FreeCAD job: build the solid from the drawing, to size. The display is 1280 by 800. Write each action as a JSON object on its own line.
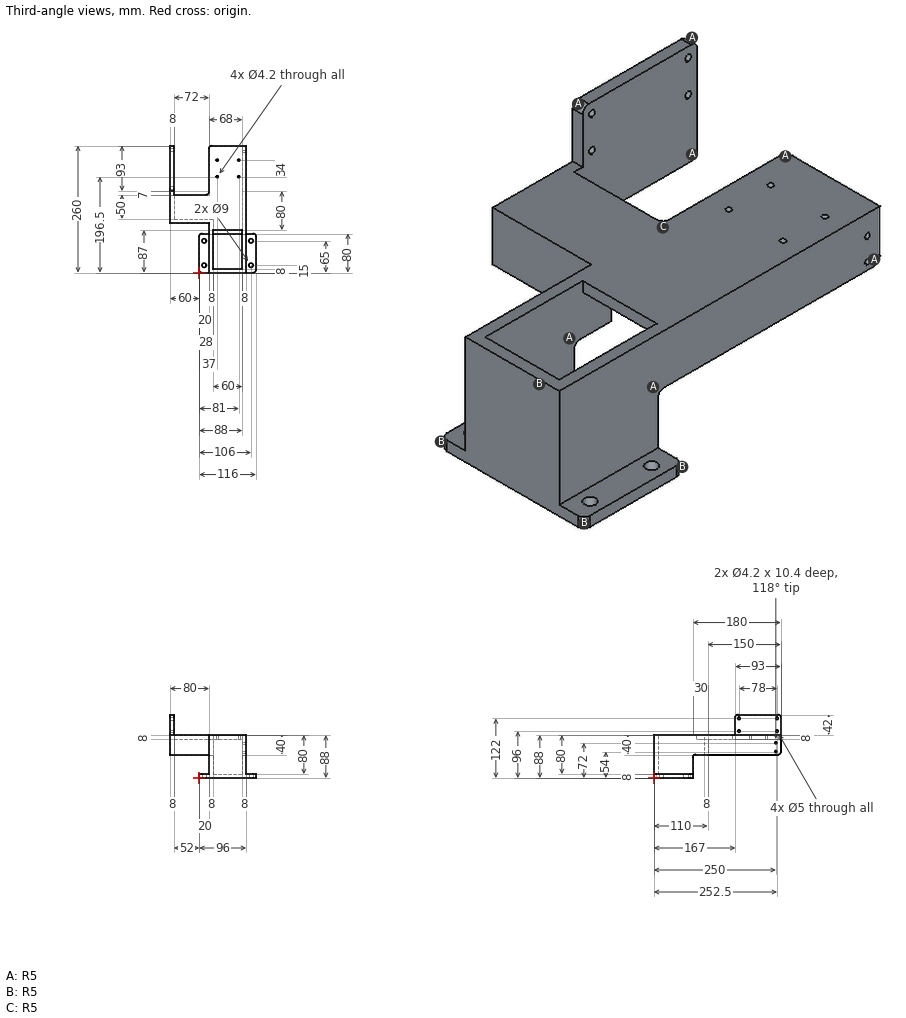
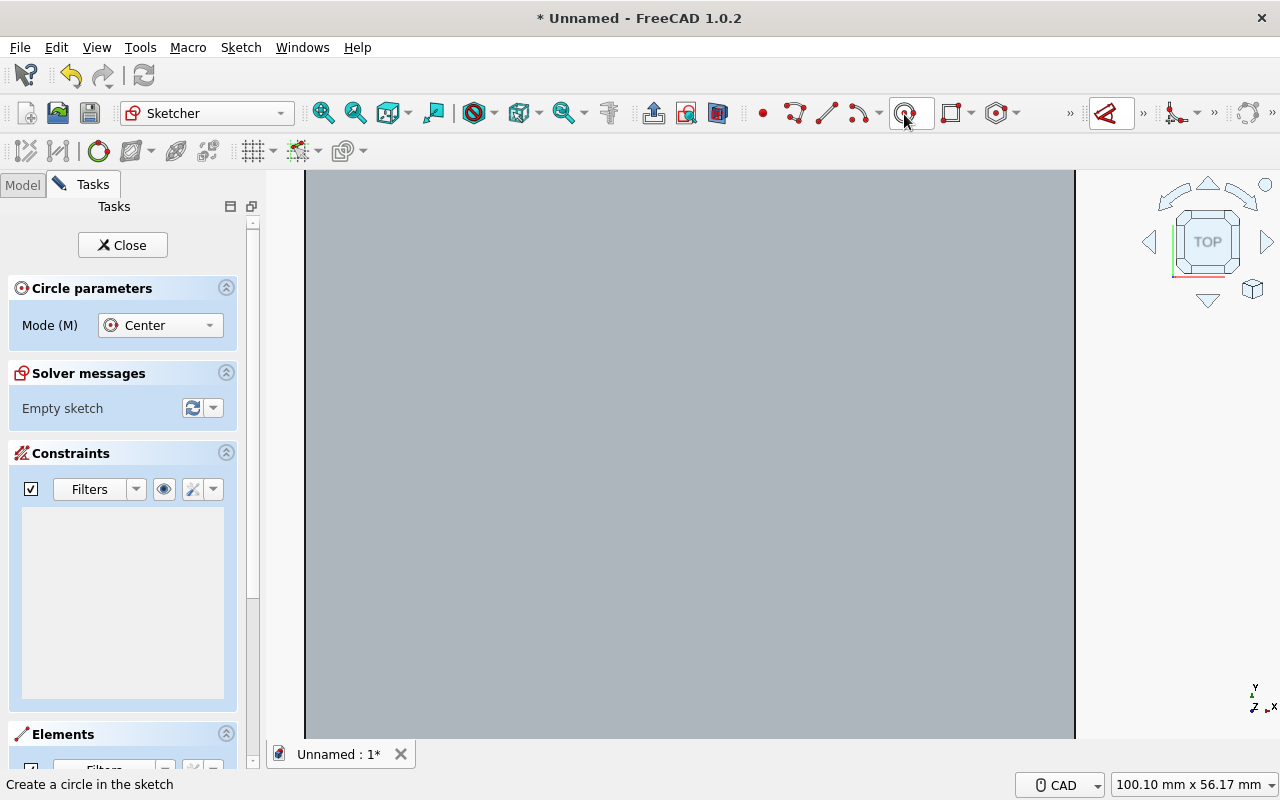
{"action": "left_click", "coordinate": [477, 626]}
{"action": "left_click", "coordinate": [493, 611]}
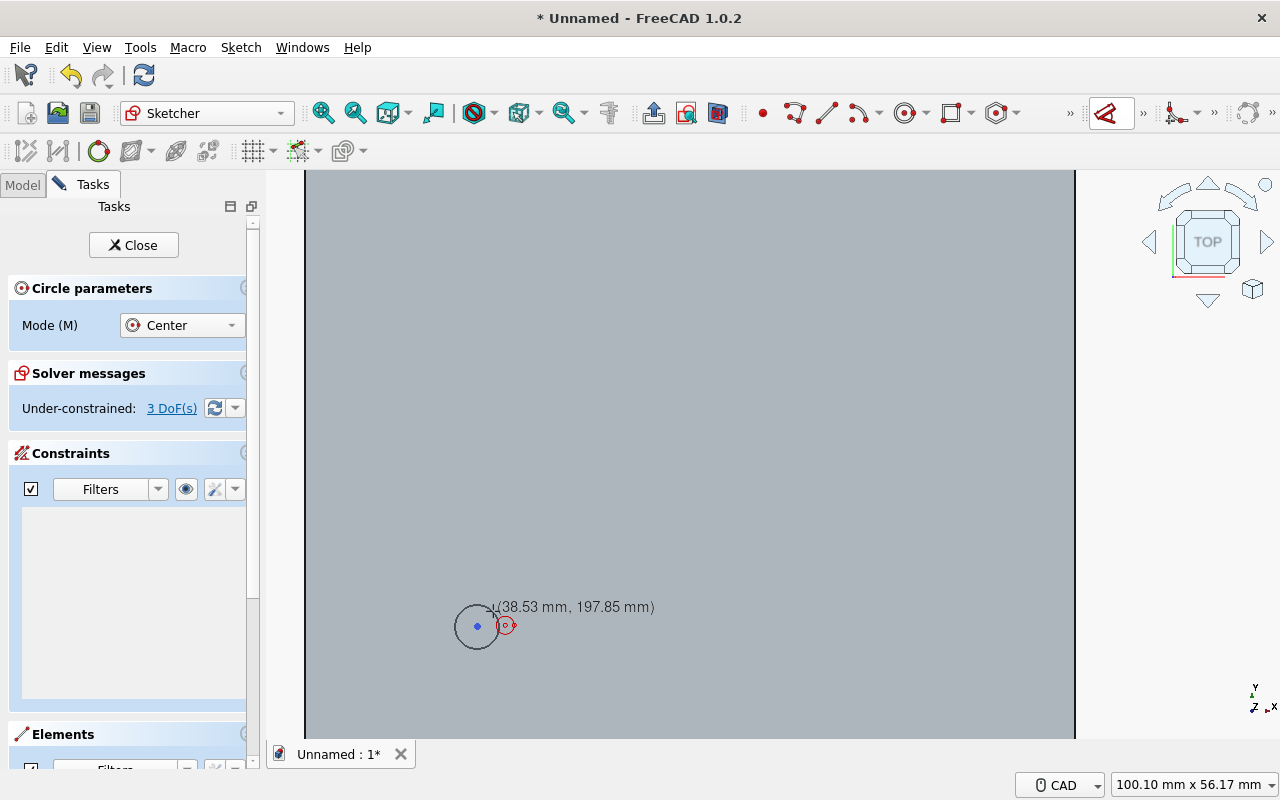
{"action": "left_click", "coordinate": [923, 626]}
{"action": "left_click", "coordinate": [938, 611]}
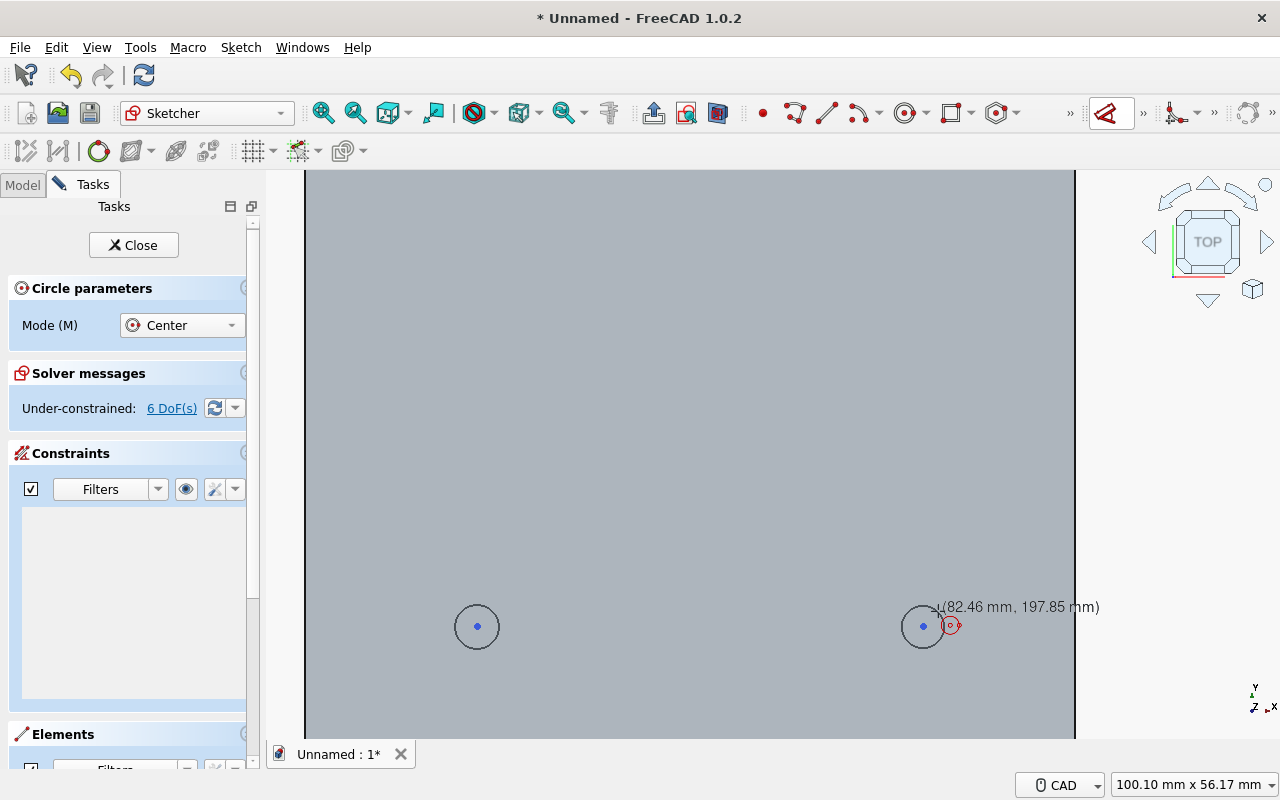
{"action": "left_click", "coordinate": [923, 281]}
{"action": "left_click", "coordinate": [938, 266]}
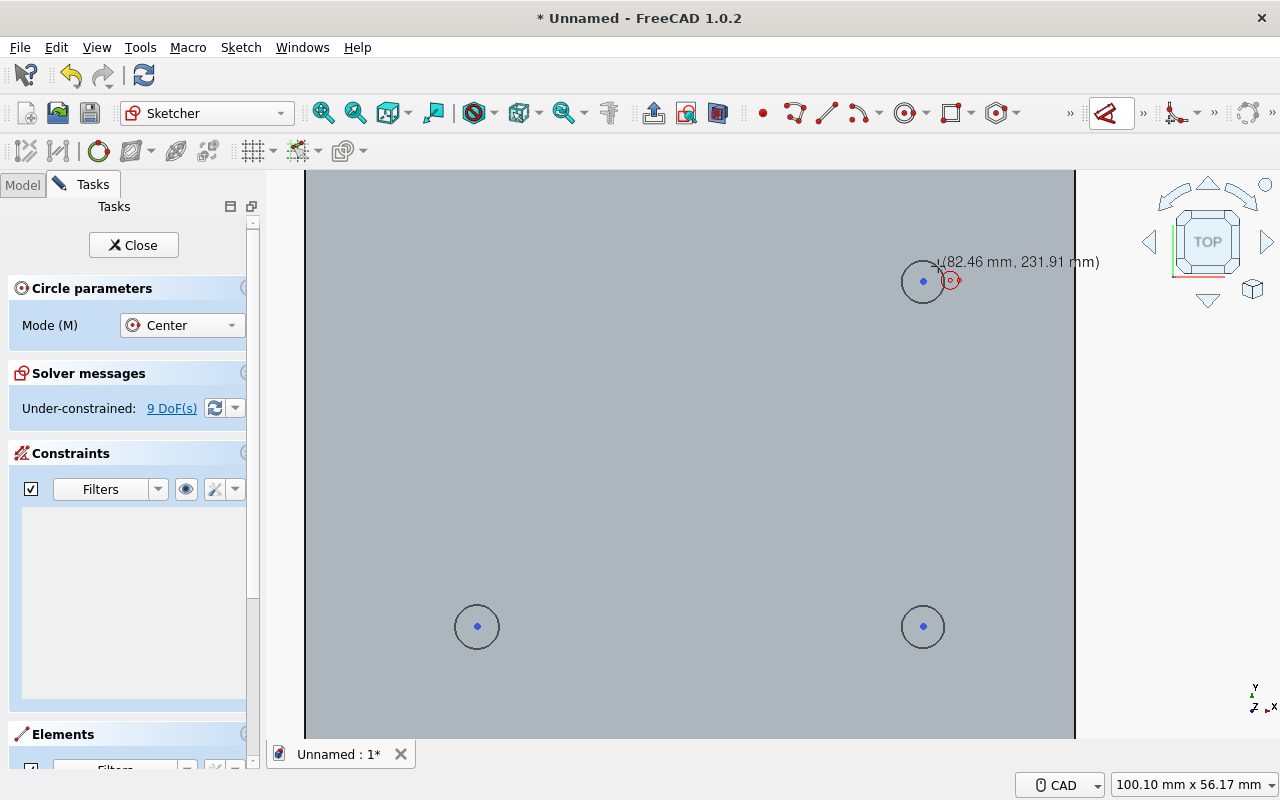
{"action": "left_click", "coordinate": [477, 281]}
{"action": "left_click", "coordinate": [493, 266]}
{"action": "key", "text": "Escape"}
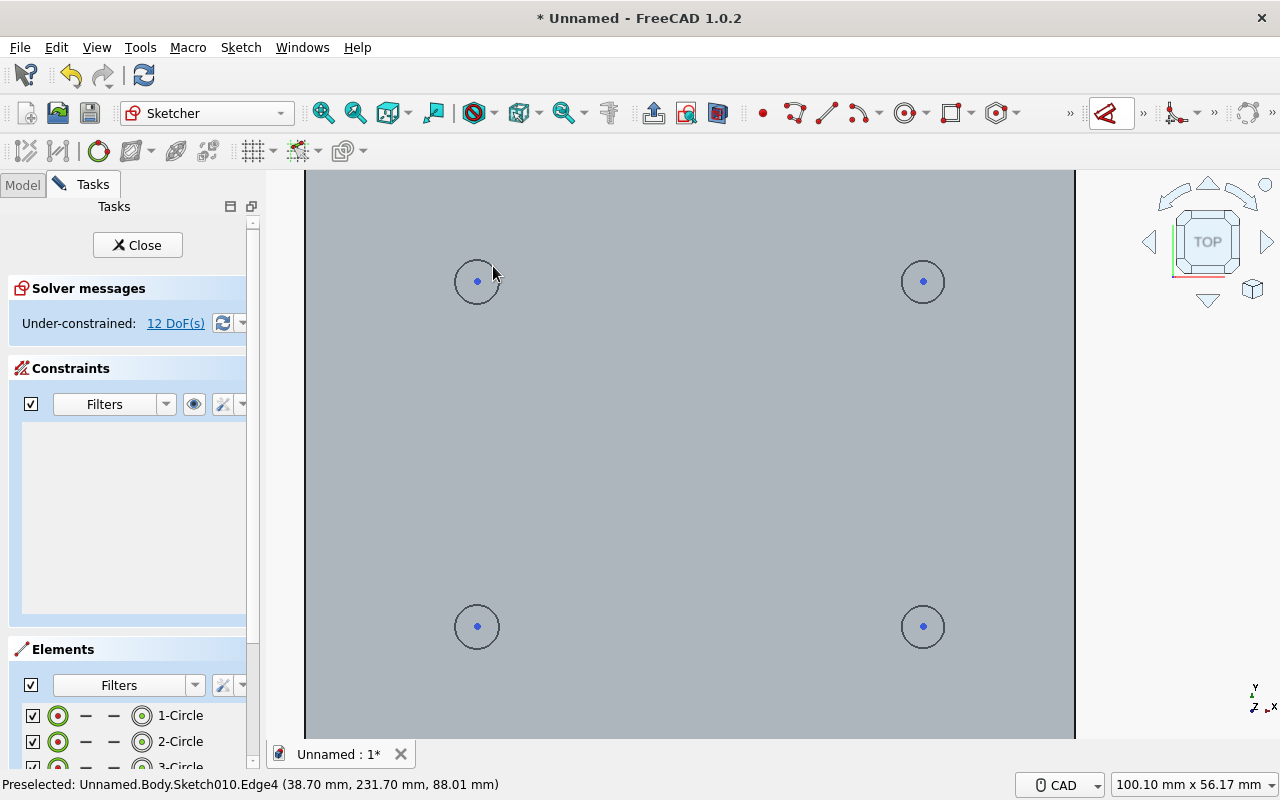
{"action": "left_click", "coordinate": [492, 611]}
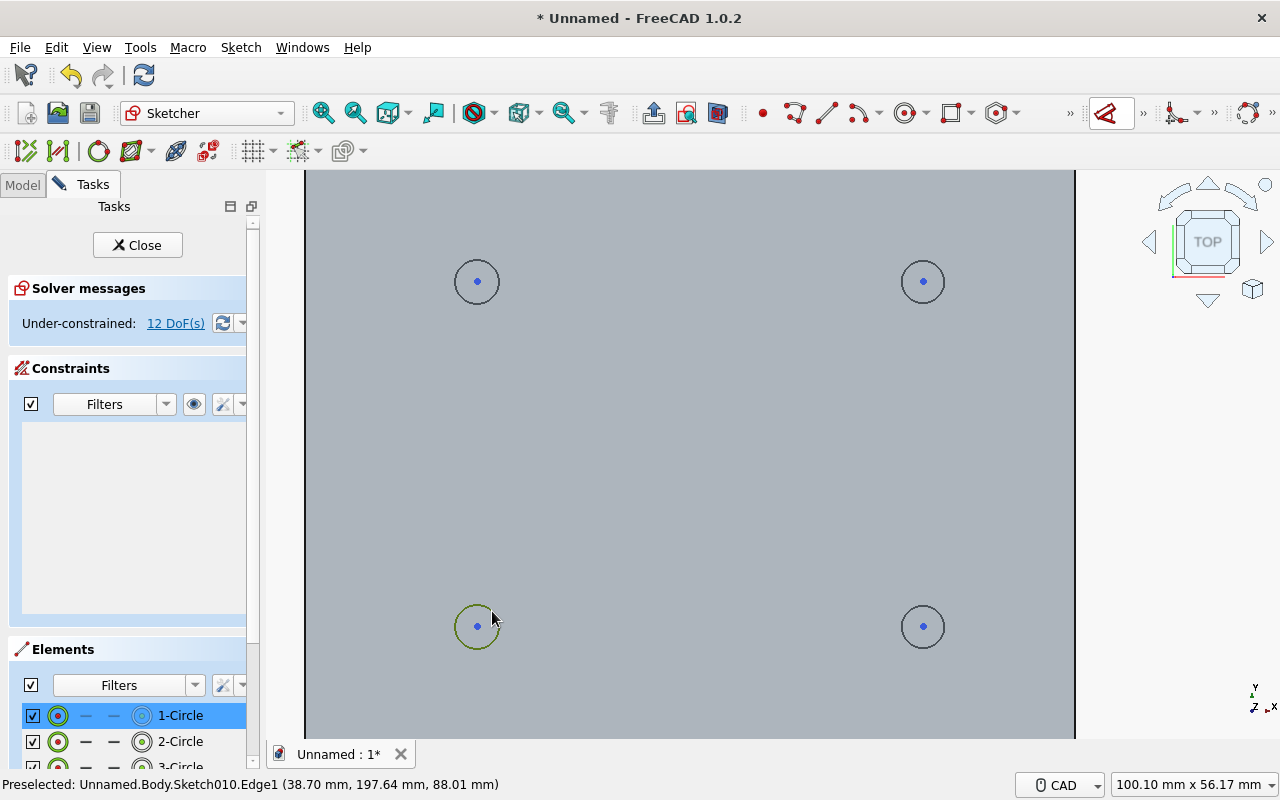
{"action": "left_click", "coordinate": [938, 612]}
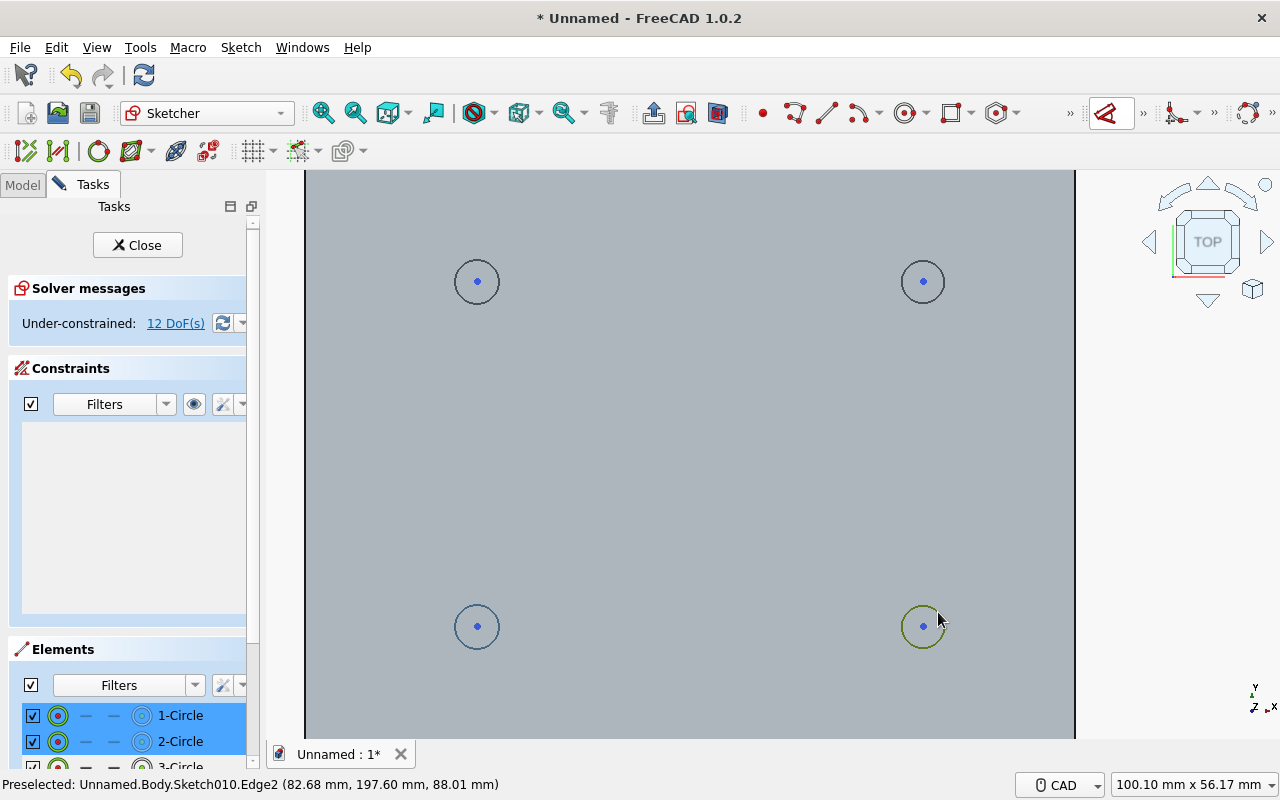
{"action": "left_click", "coordinate": [938, 267]}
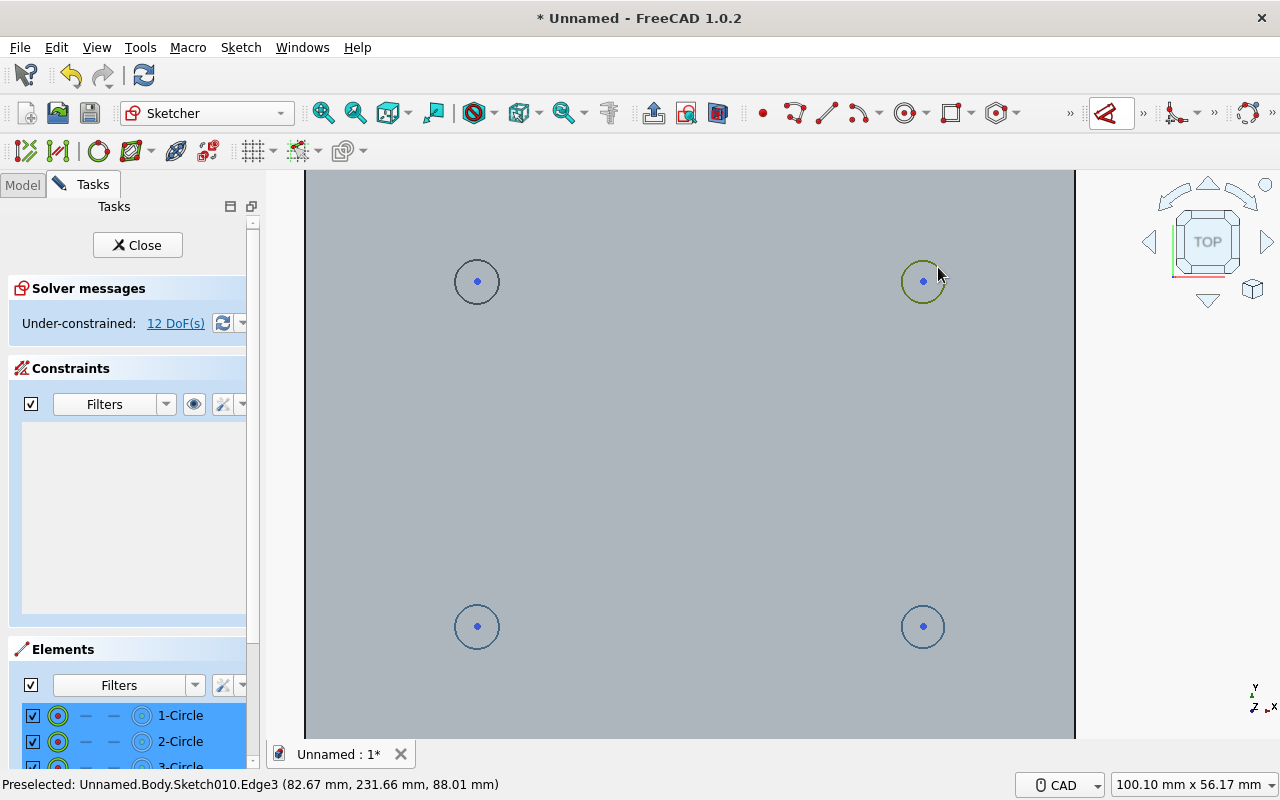
{"action": "left_click", "coordinate": [492, 266]}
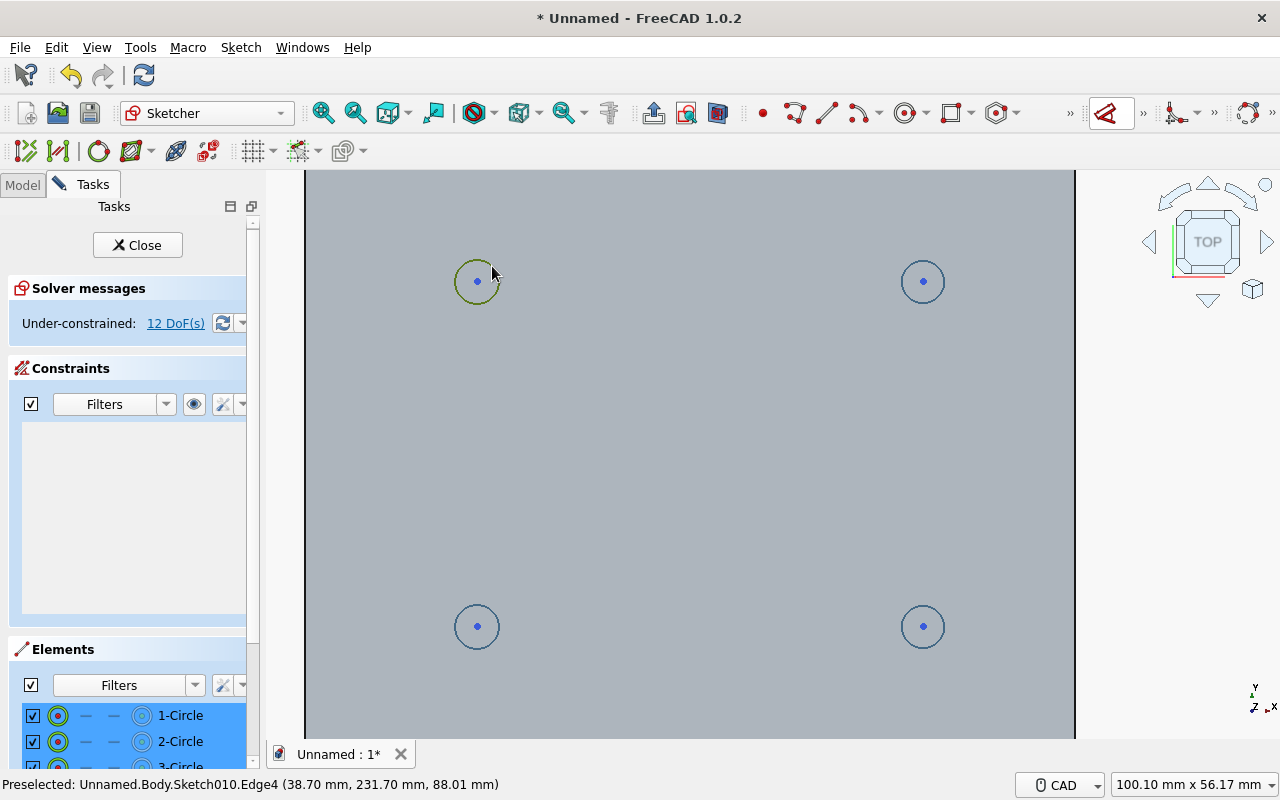
{"action": "key", "text": "e"}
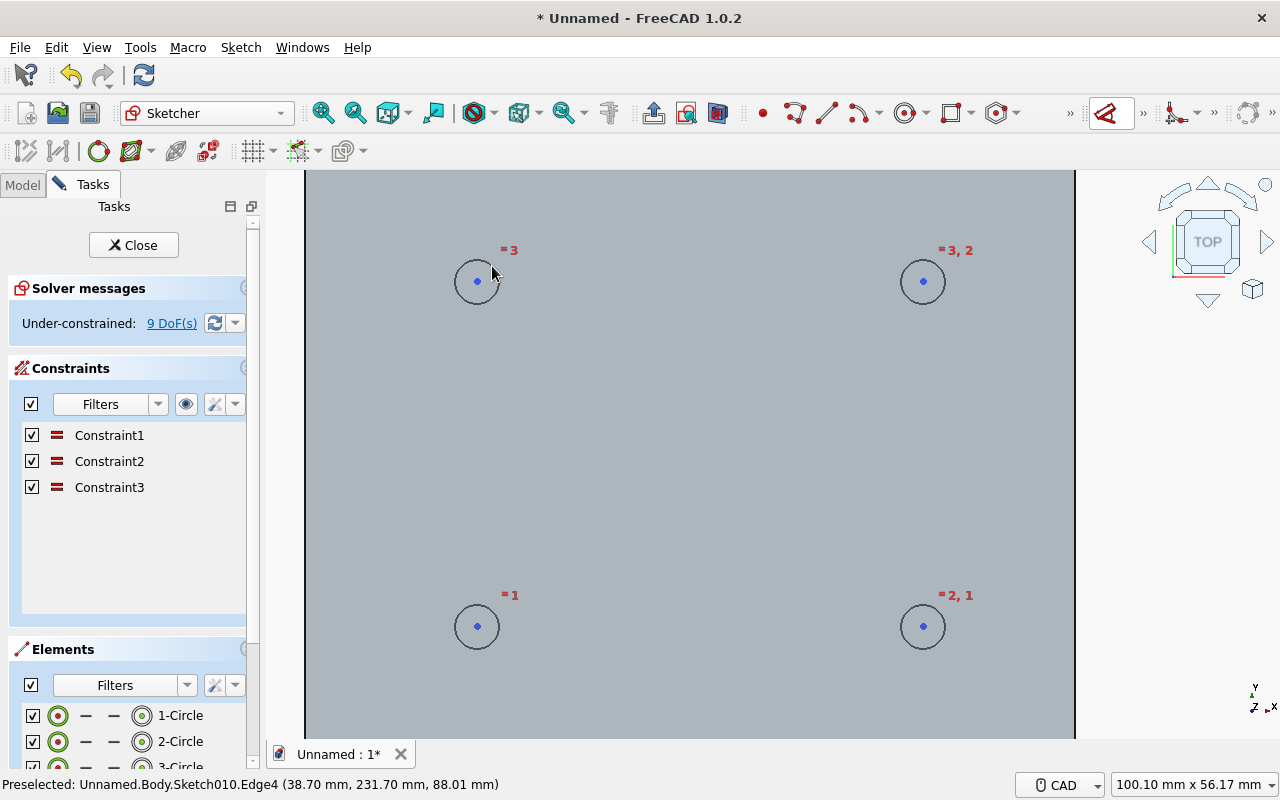
{"action": "left_click", "coordinate": [477, 627]}